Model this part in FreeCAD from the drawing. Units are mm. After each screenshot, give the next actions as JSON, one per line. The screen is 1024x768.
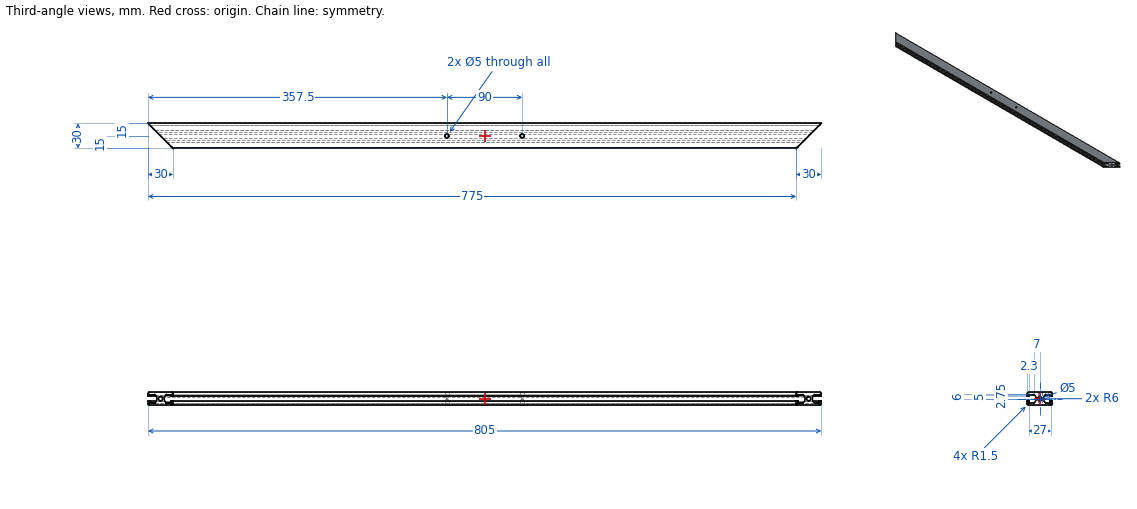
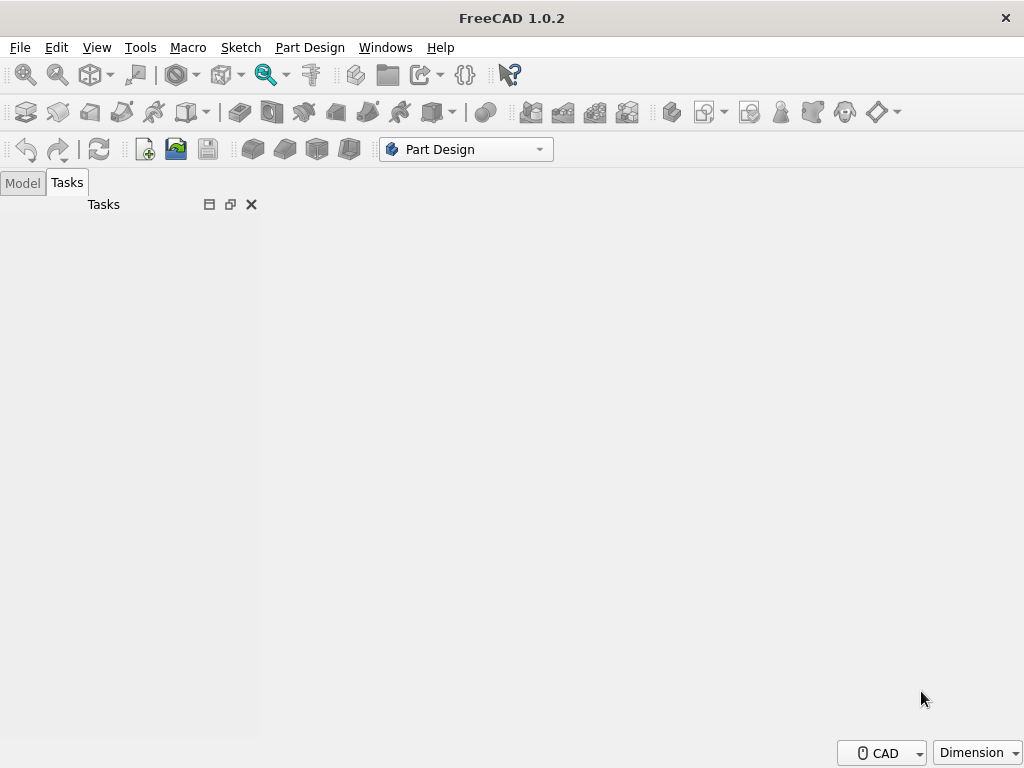
{"action": "left_click", "coordinate": [144, 150]}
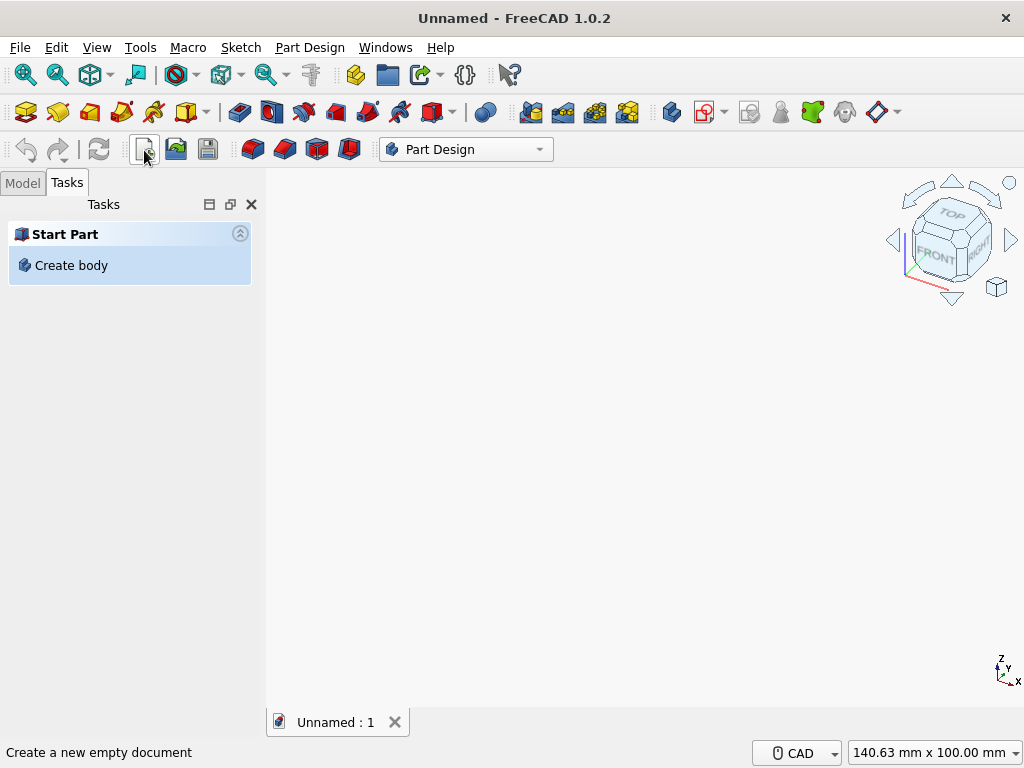
{"action": "left_click", "coordinate": [672, 112]}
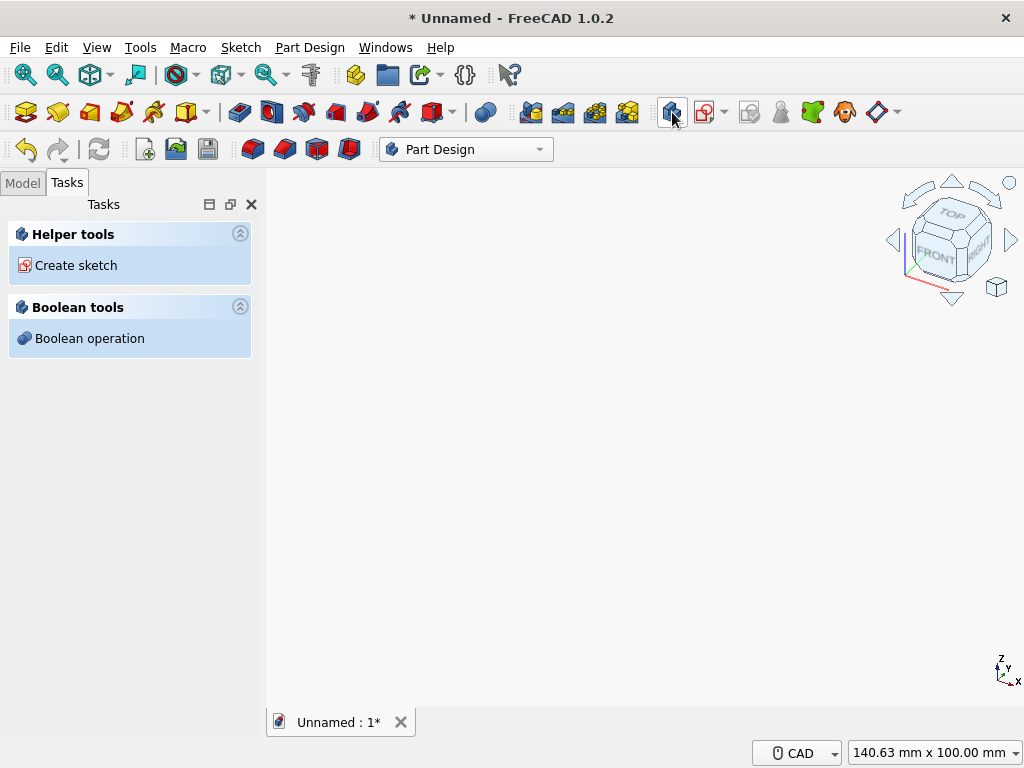
{"action": "left_click", "coordinate": [23, 182]}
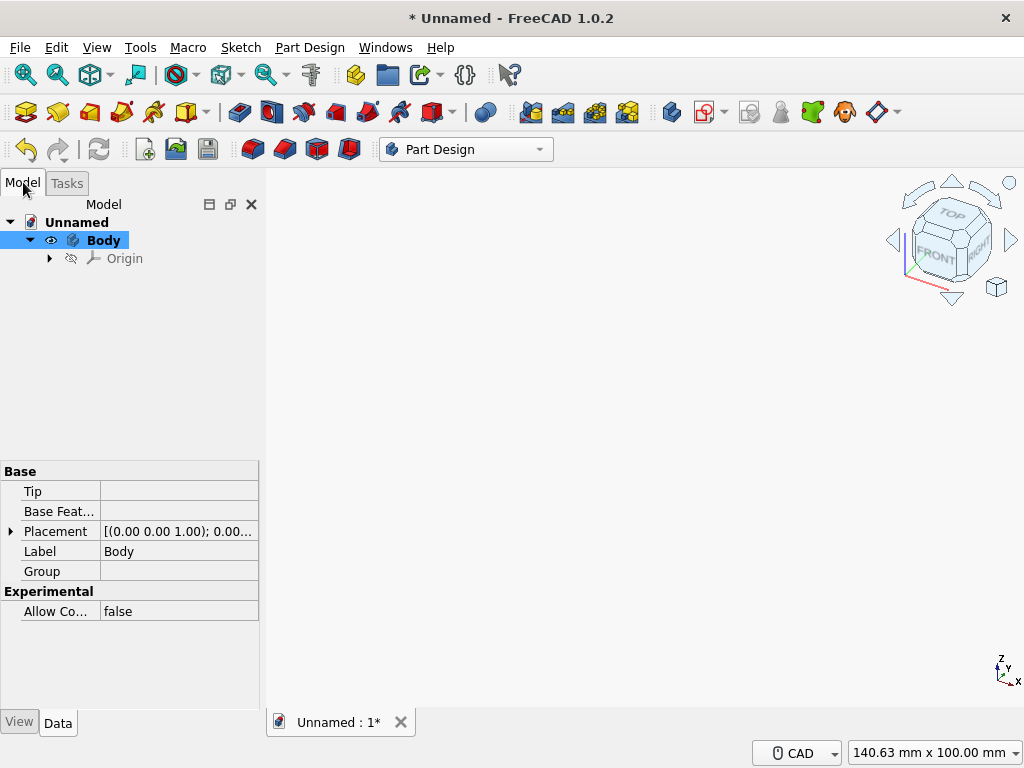
{"action": "left_click", "coordinate": [50, 258]}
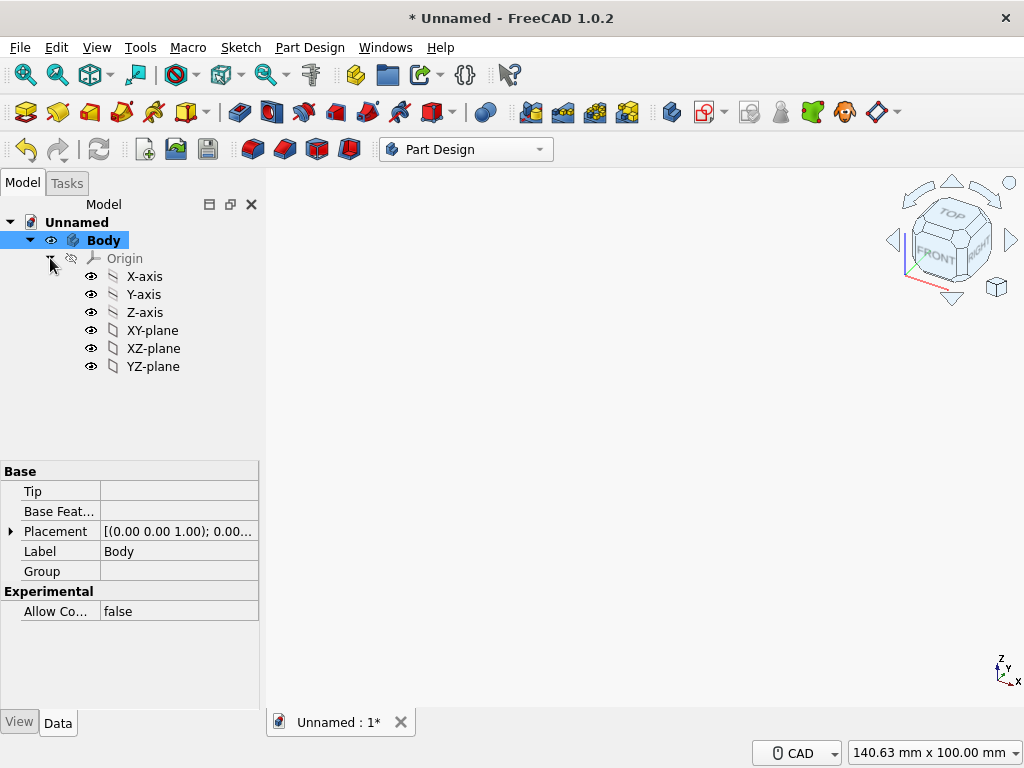
{"action": "left_click", "coordinate": [136, 366]}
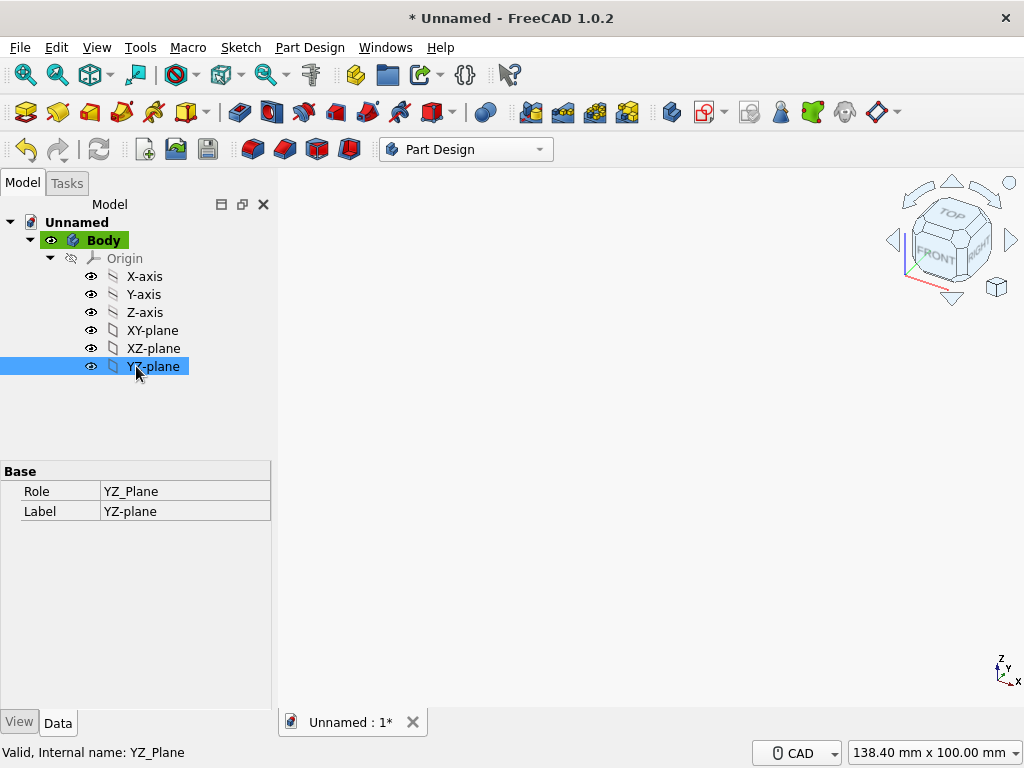
{"action": "left_click", "coordinate": [878, 112]}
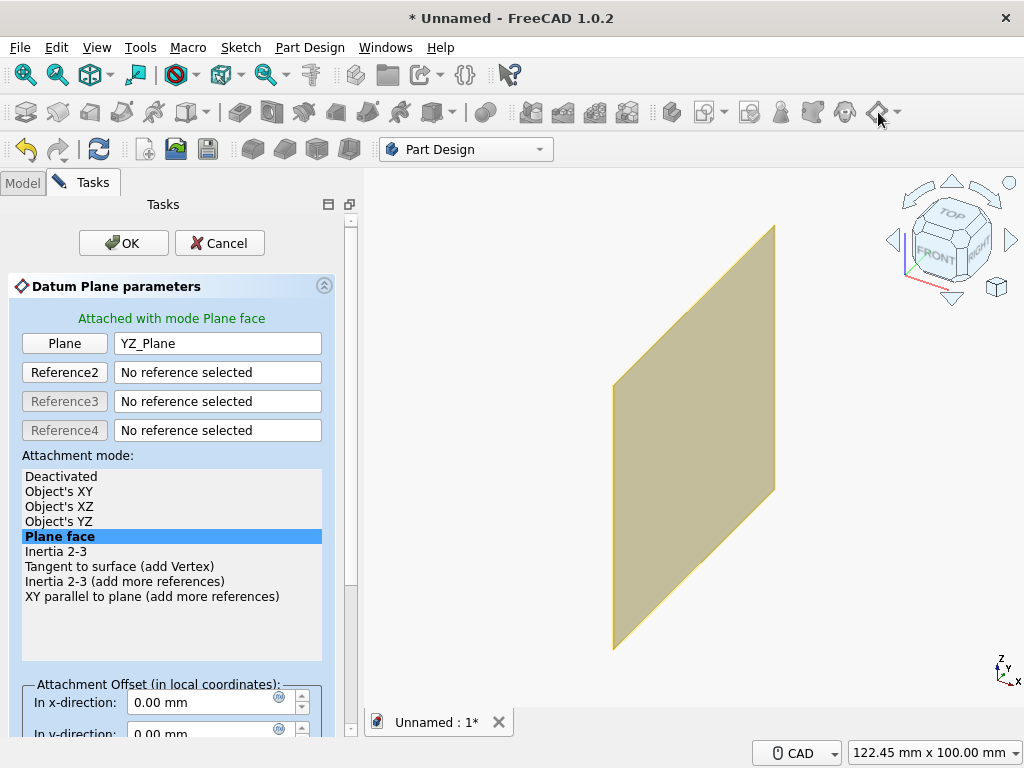
{"action": "scroll", "coordinate": [351, 475], "scroll_direction": "down", "scroll_amount": 2}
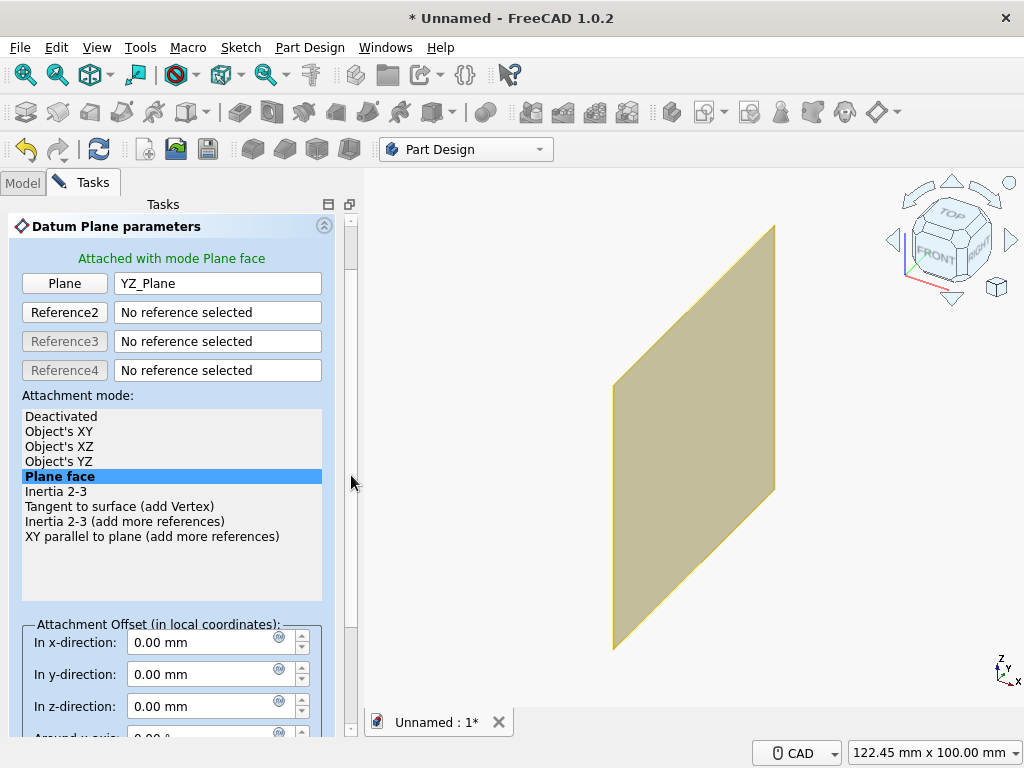
{"action": "triple_click", "coordinate": [210, 646]}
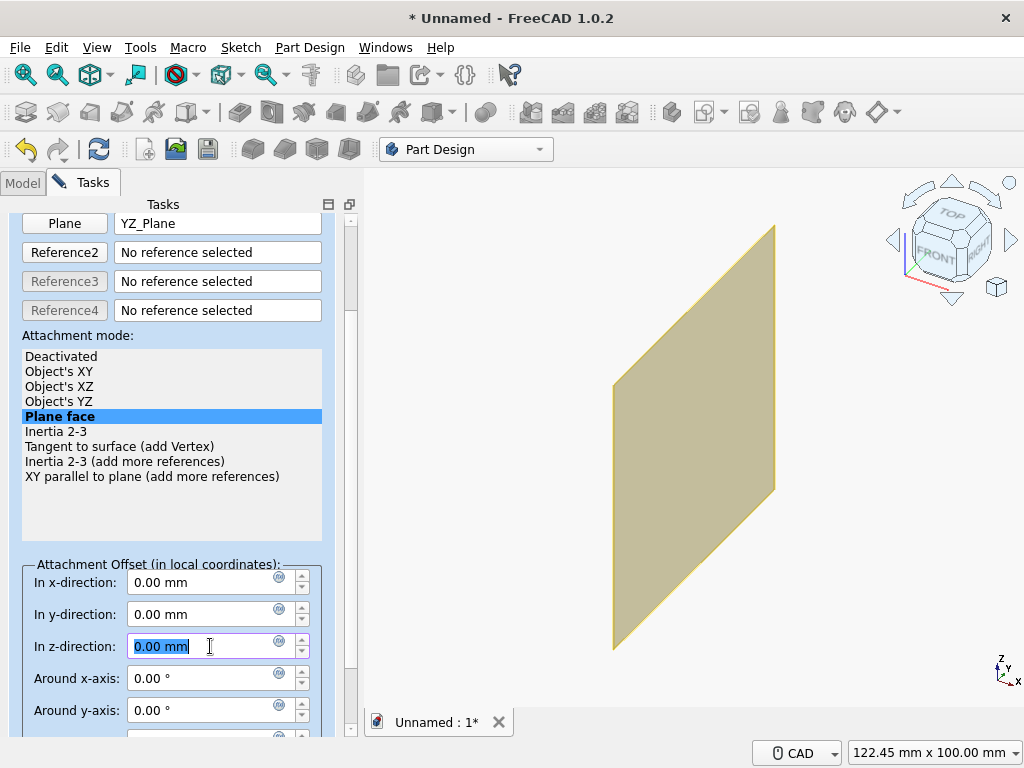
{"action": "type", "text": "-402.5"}
{"action": "key", "text": "Tab"}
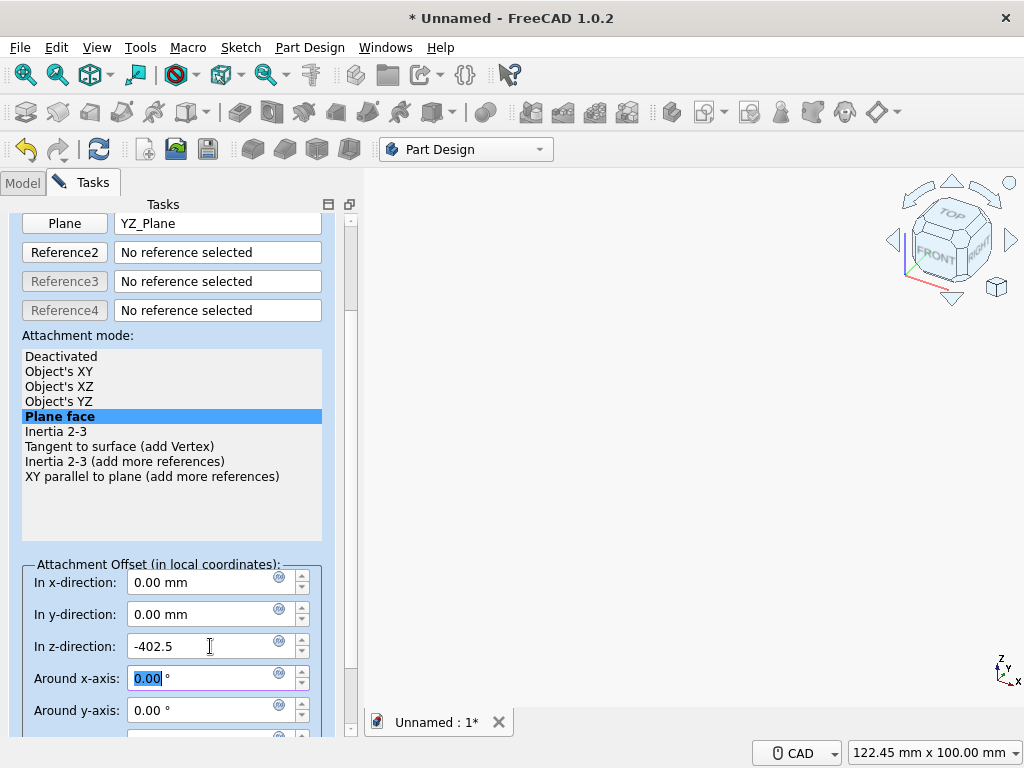
{"action": "scroll", "coordinate": [351, 475], "scroll_direction": "up", "scroll_amount": 3}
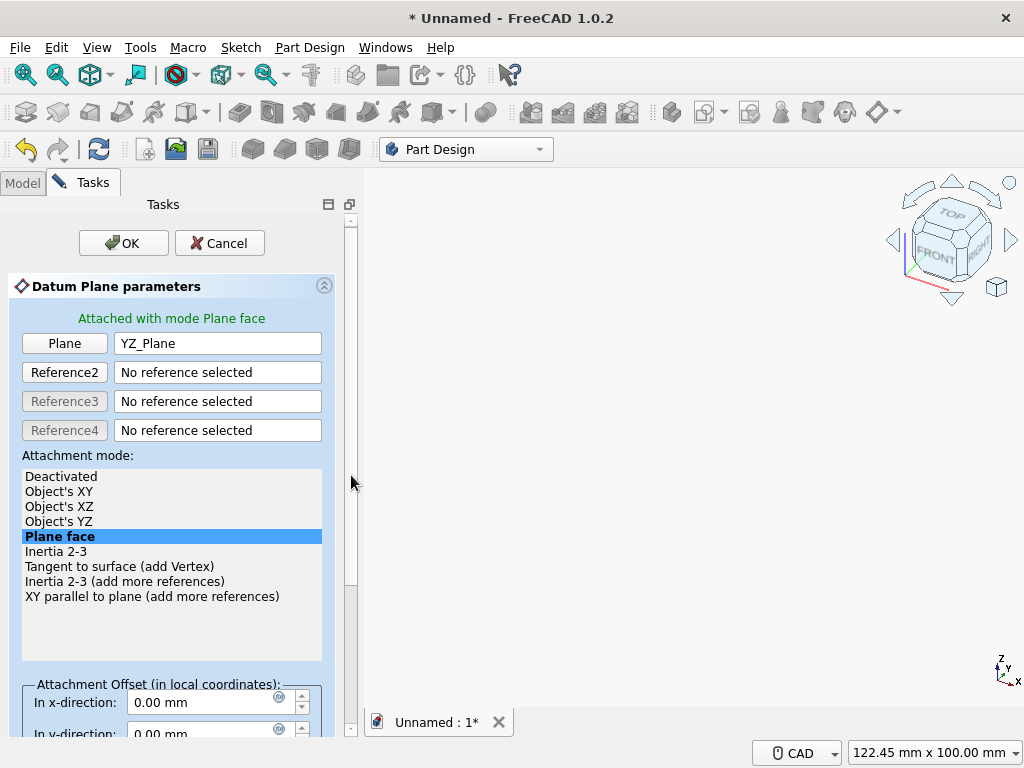
{"action": "left_click", "coordinate": [124, 243]}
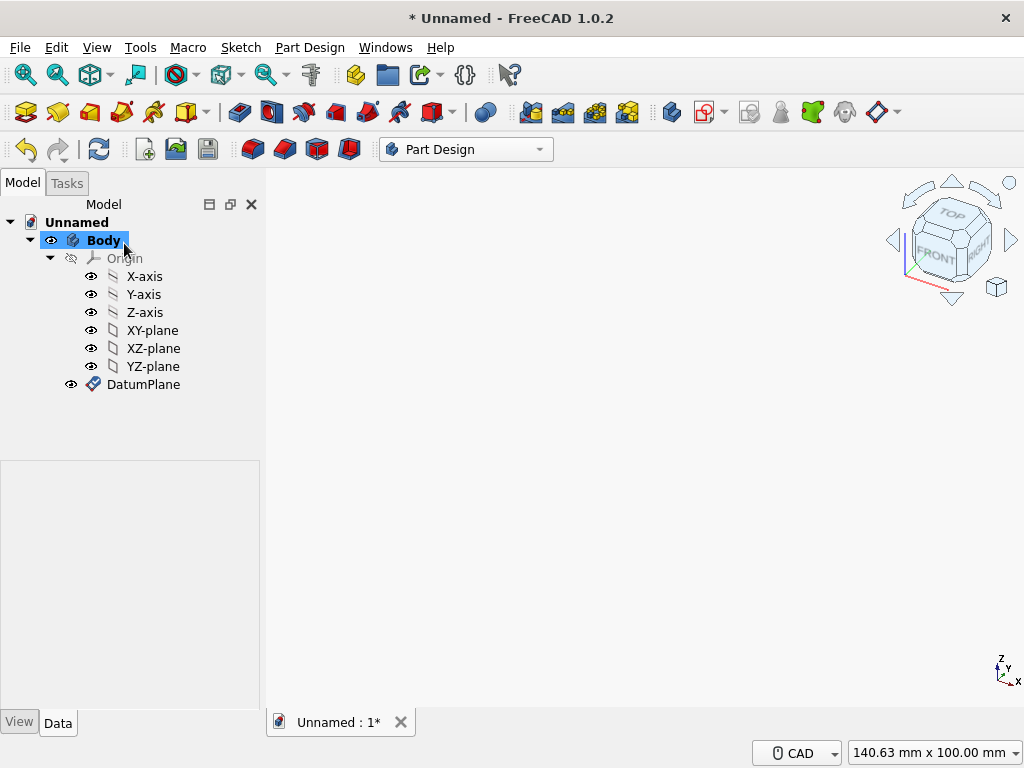
{"action": "left_click", "coordinate": [116, 384]}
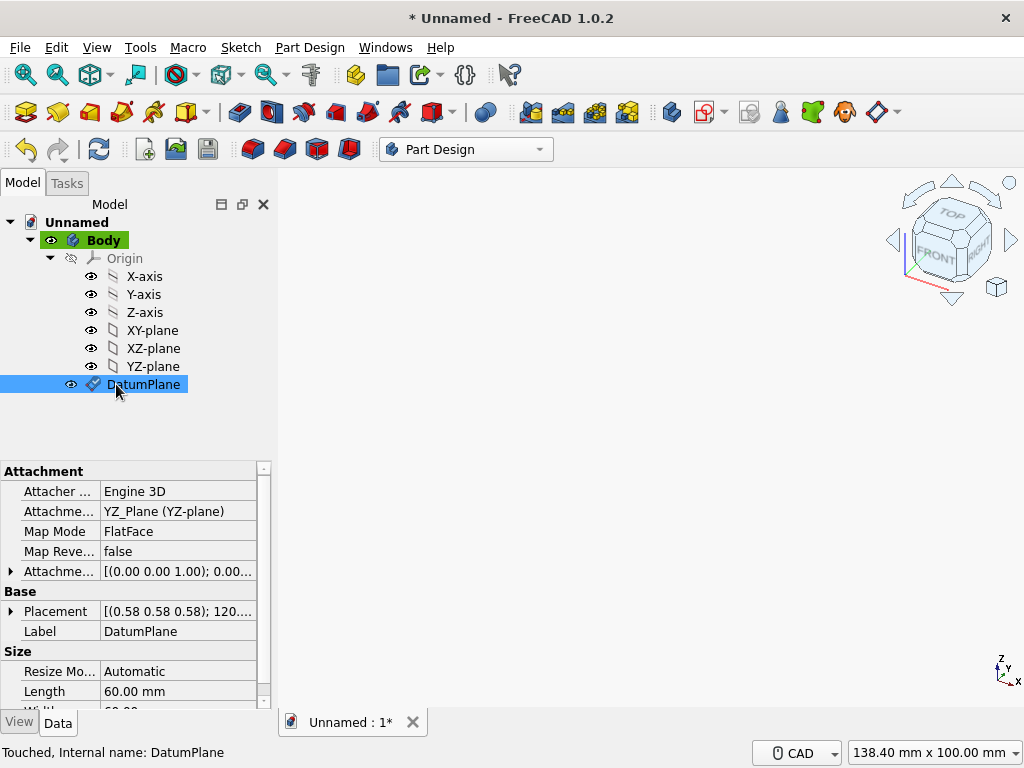
{"action": "left_click", "coordinate": [704, 112]}